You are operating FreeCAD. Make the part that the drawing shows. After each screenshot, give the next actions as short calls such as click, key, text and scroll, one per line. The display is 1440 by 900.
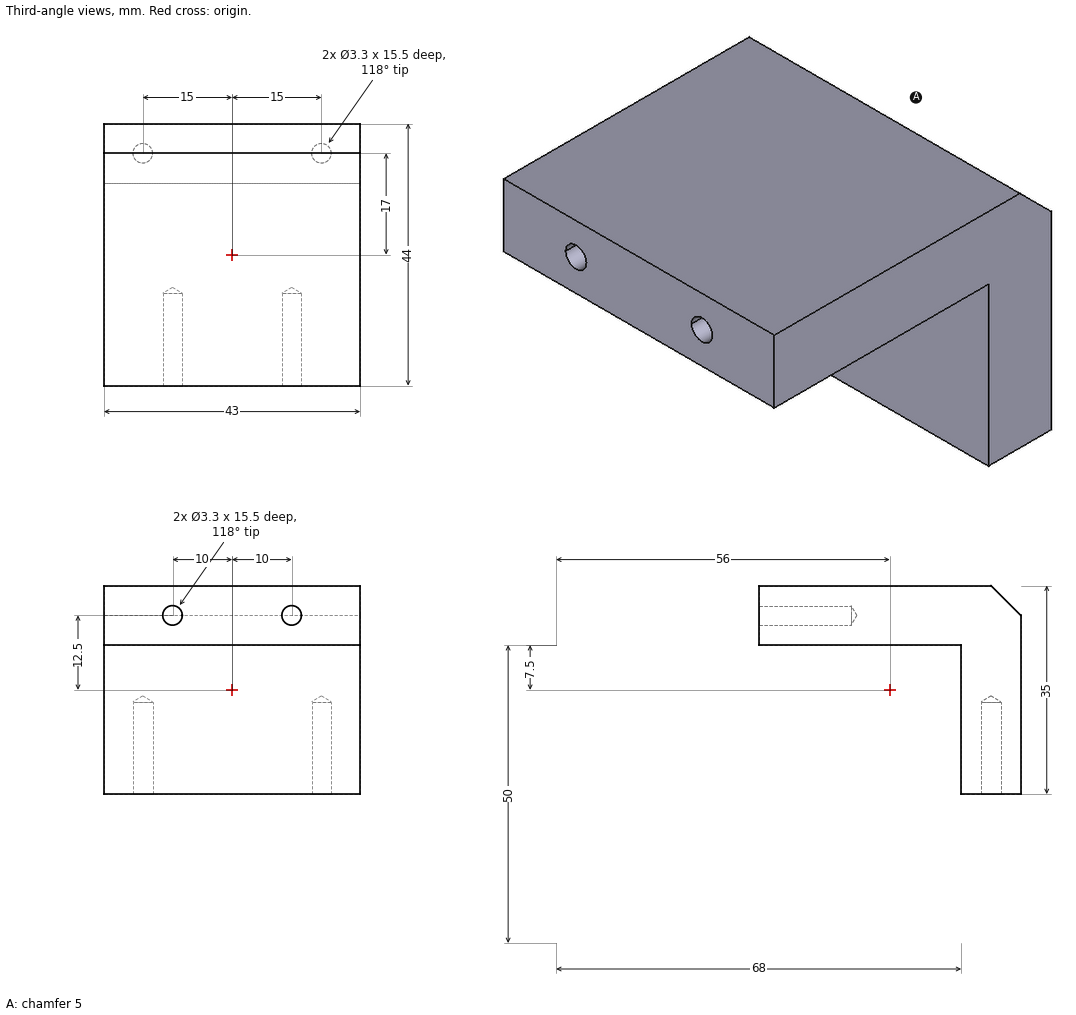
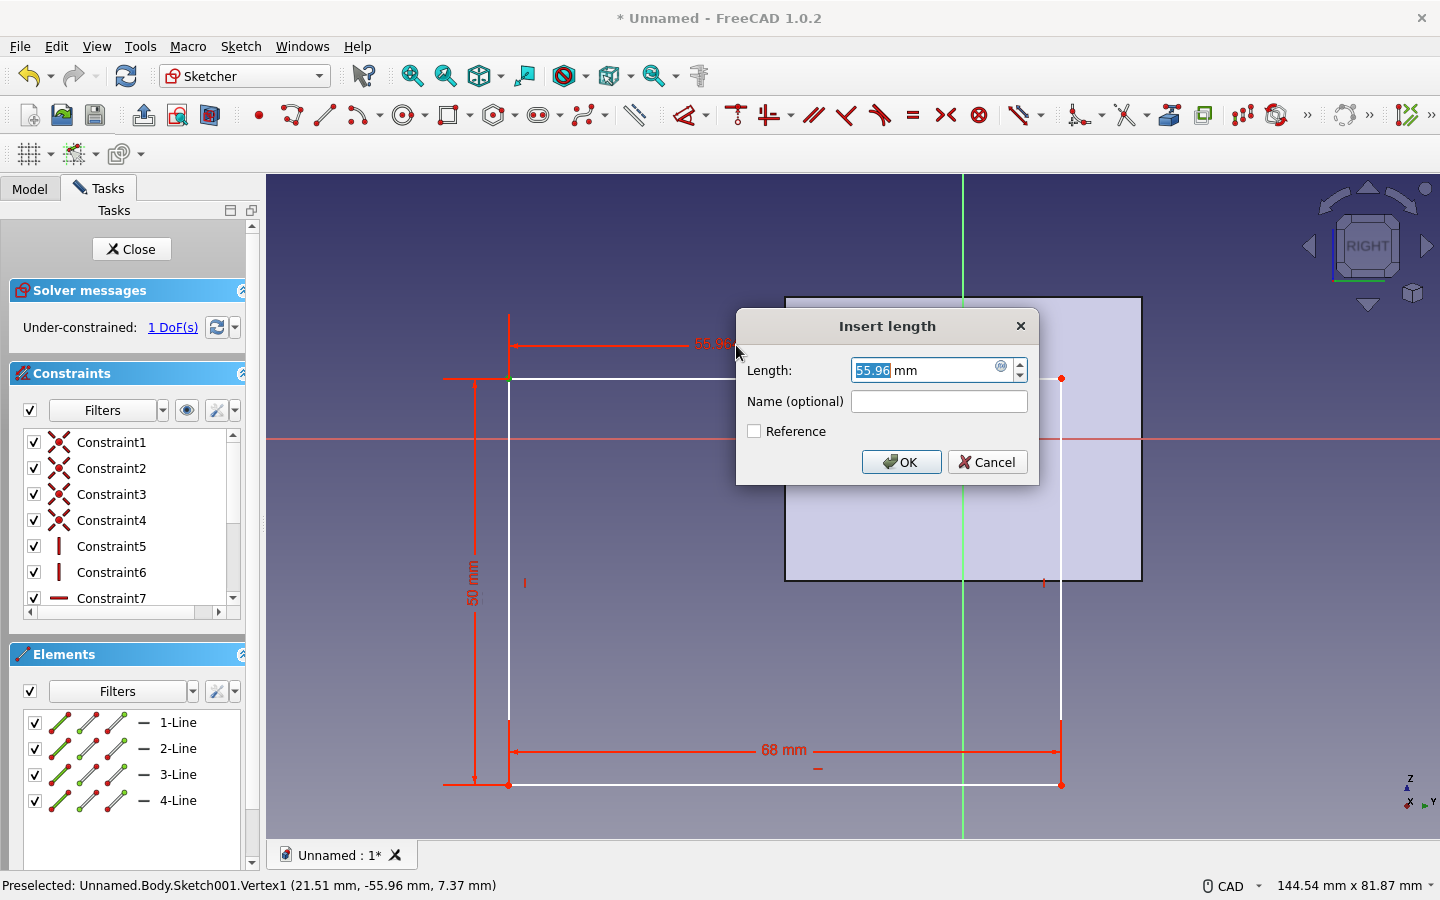
text(56)
key(Return)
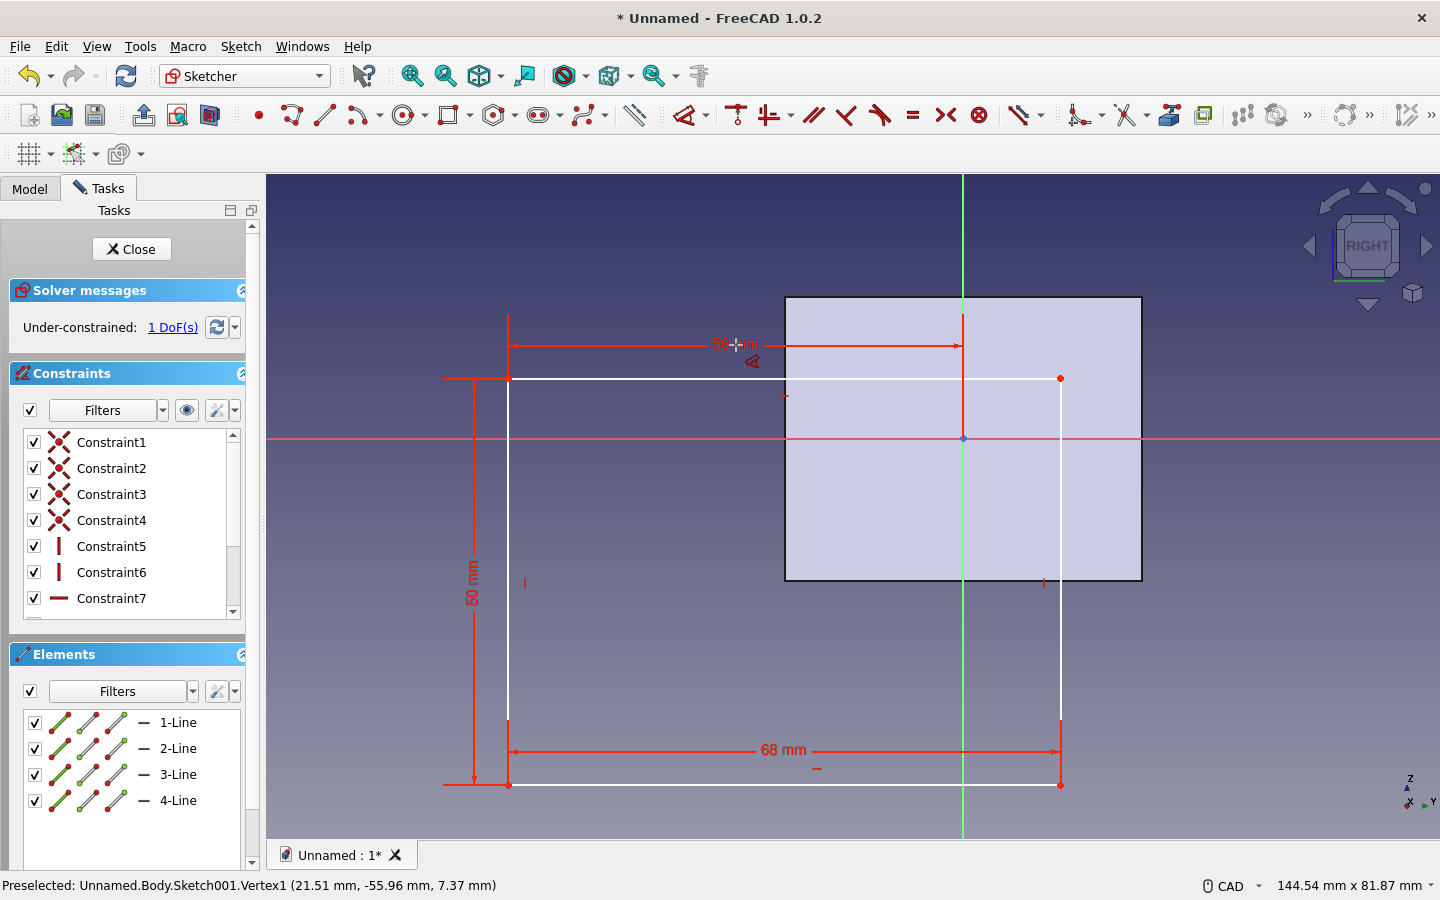
click(508, 379)
click(474, 409)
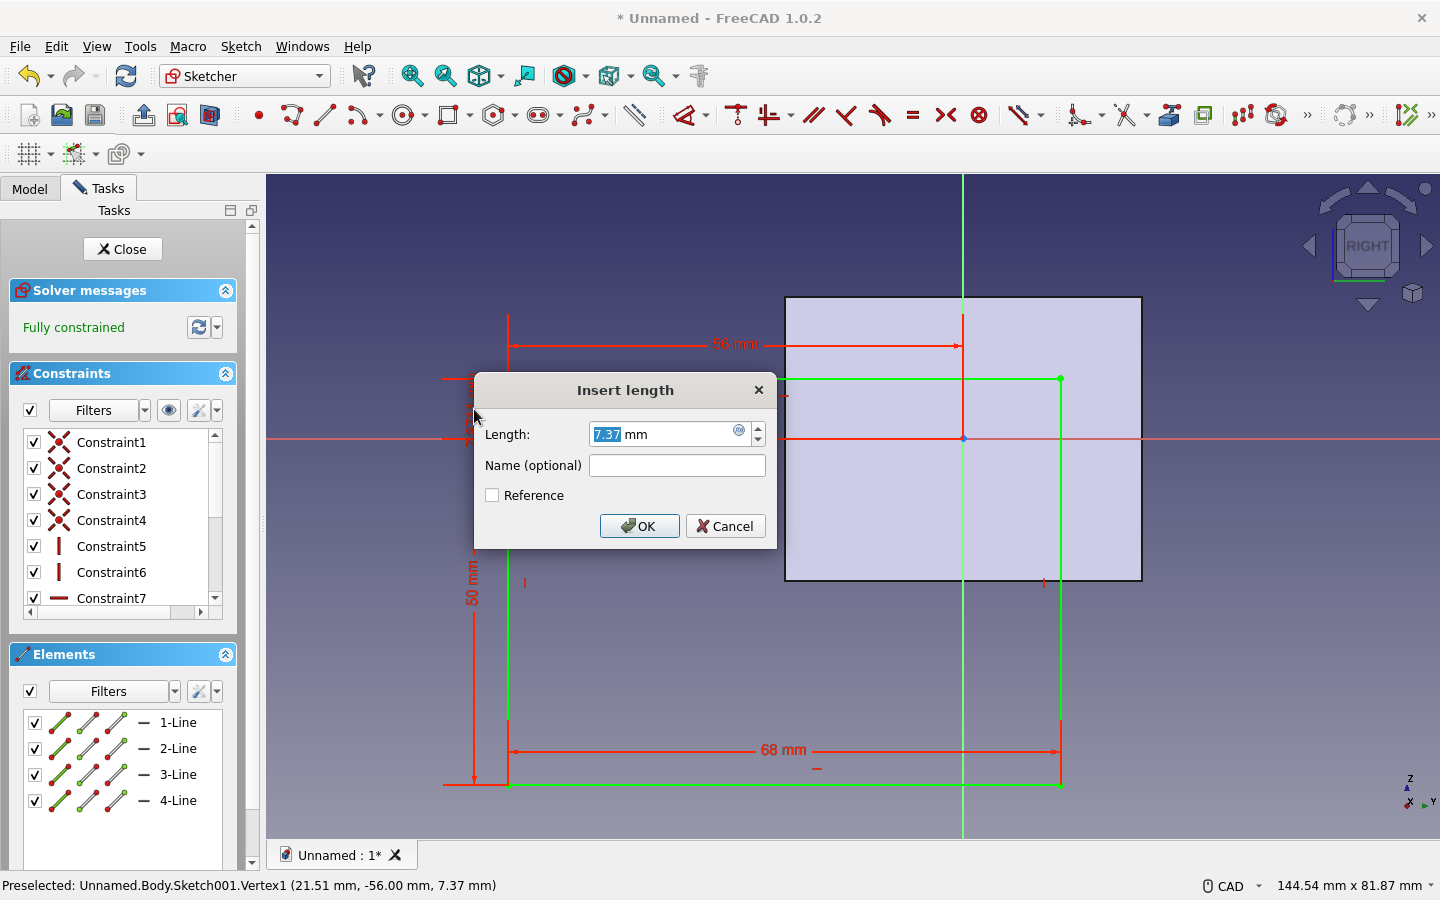
text(7.5)
key(Return)
key(Escape)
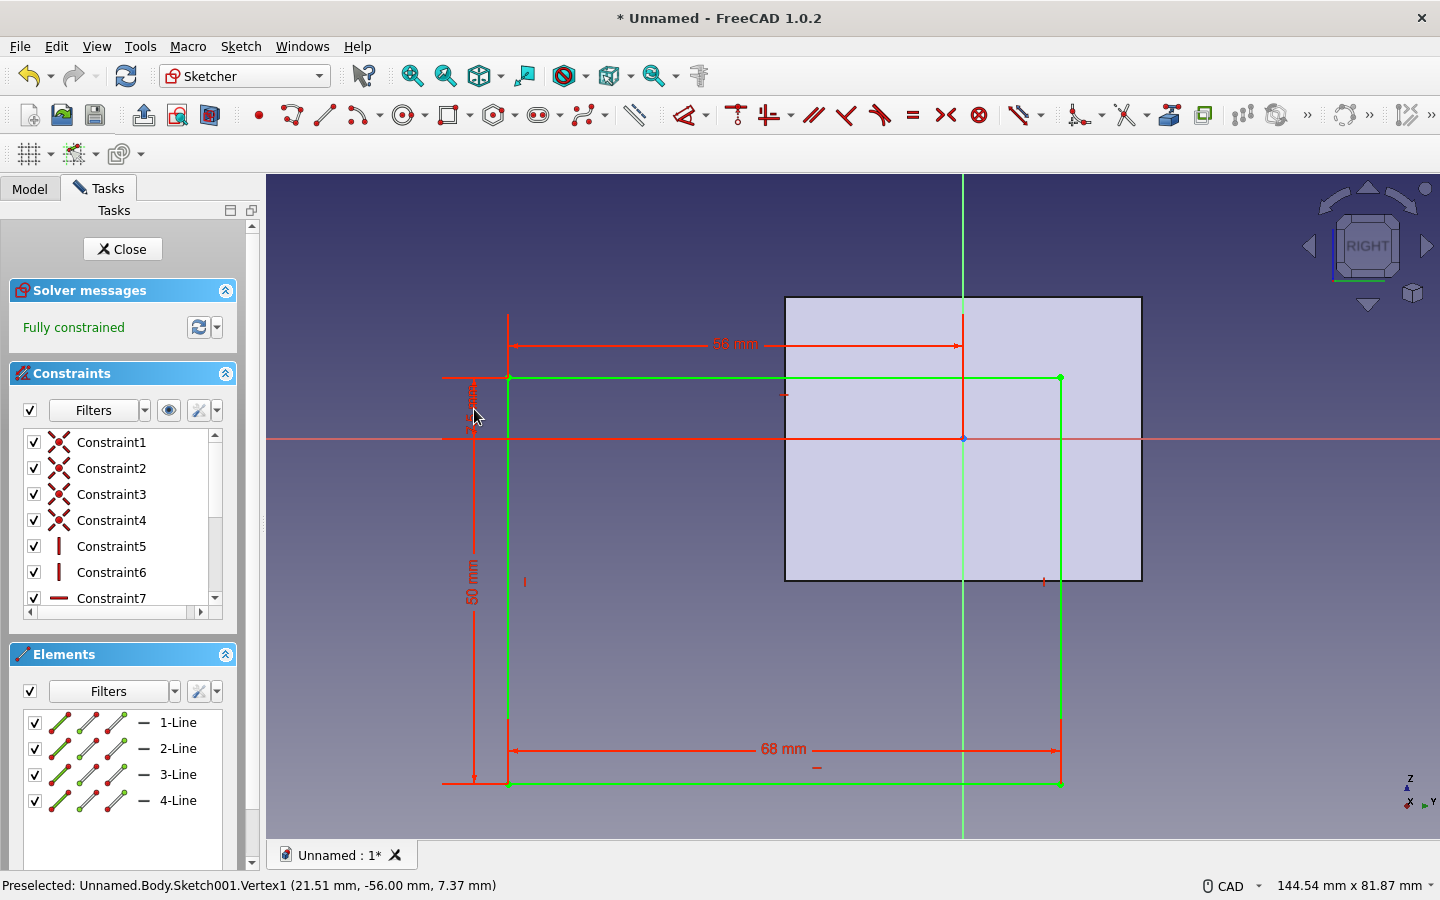
click(123, 249)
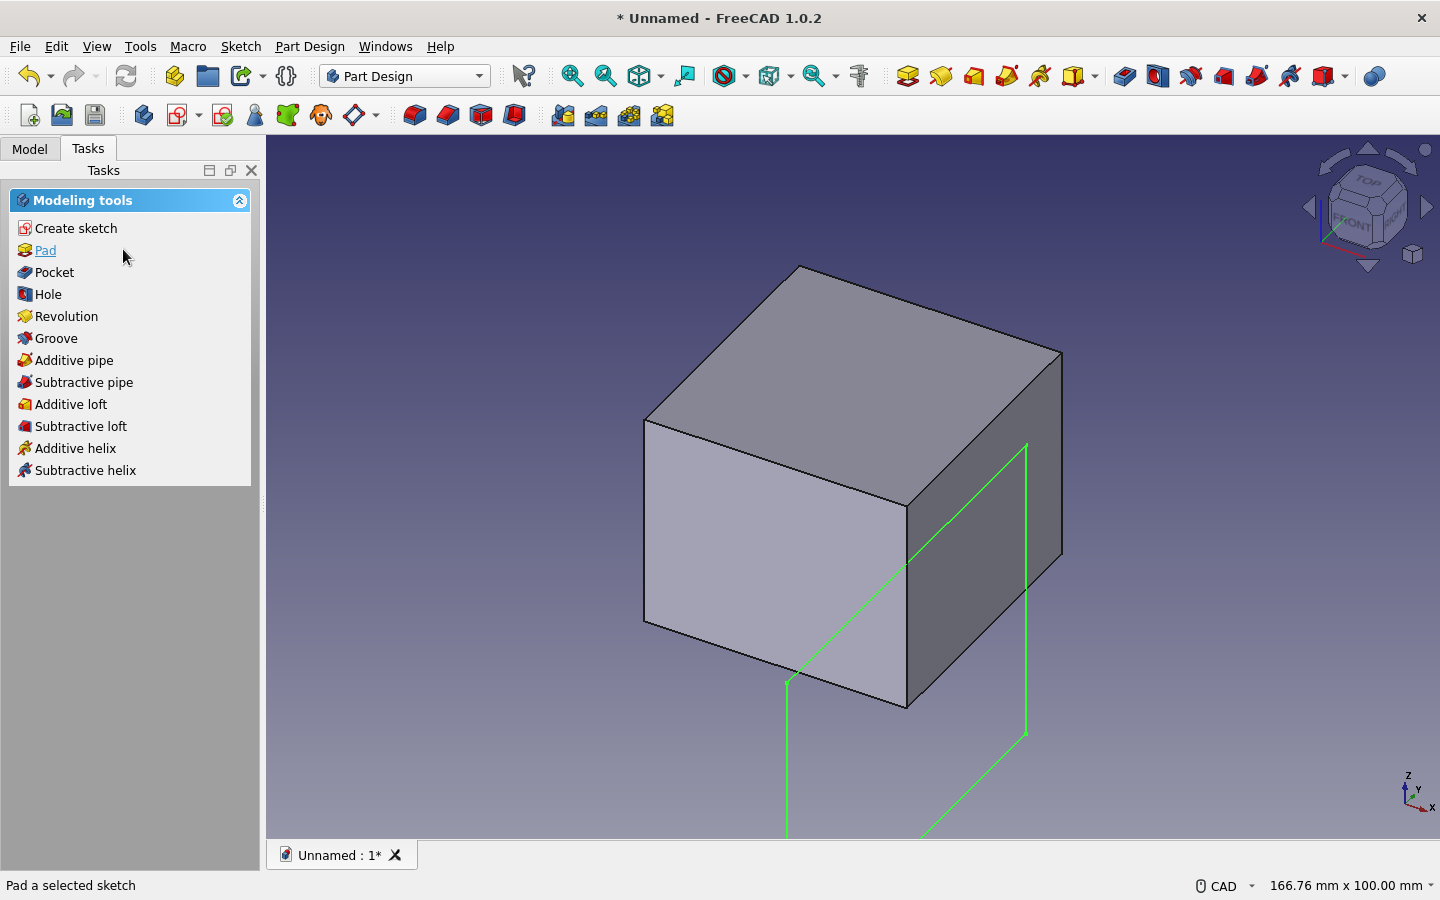
click(1125, 76)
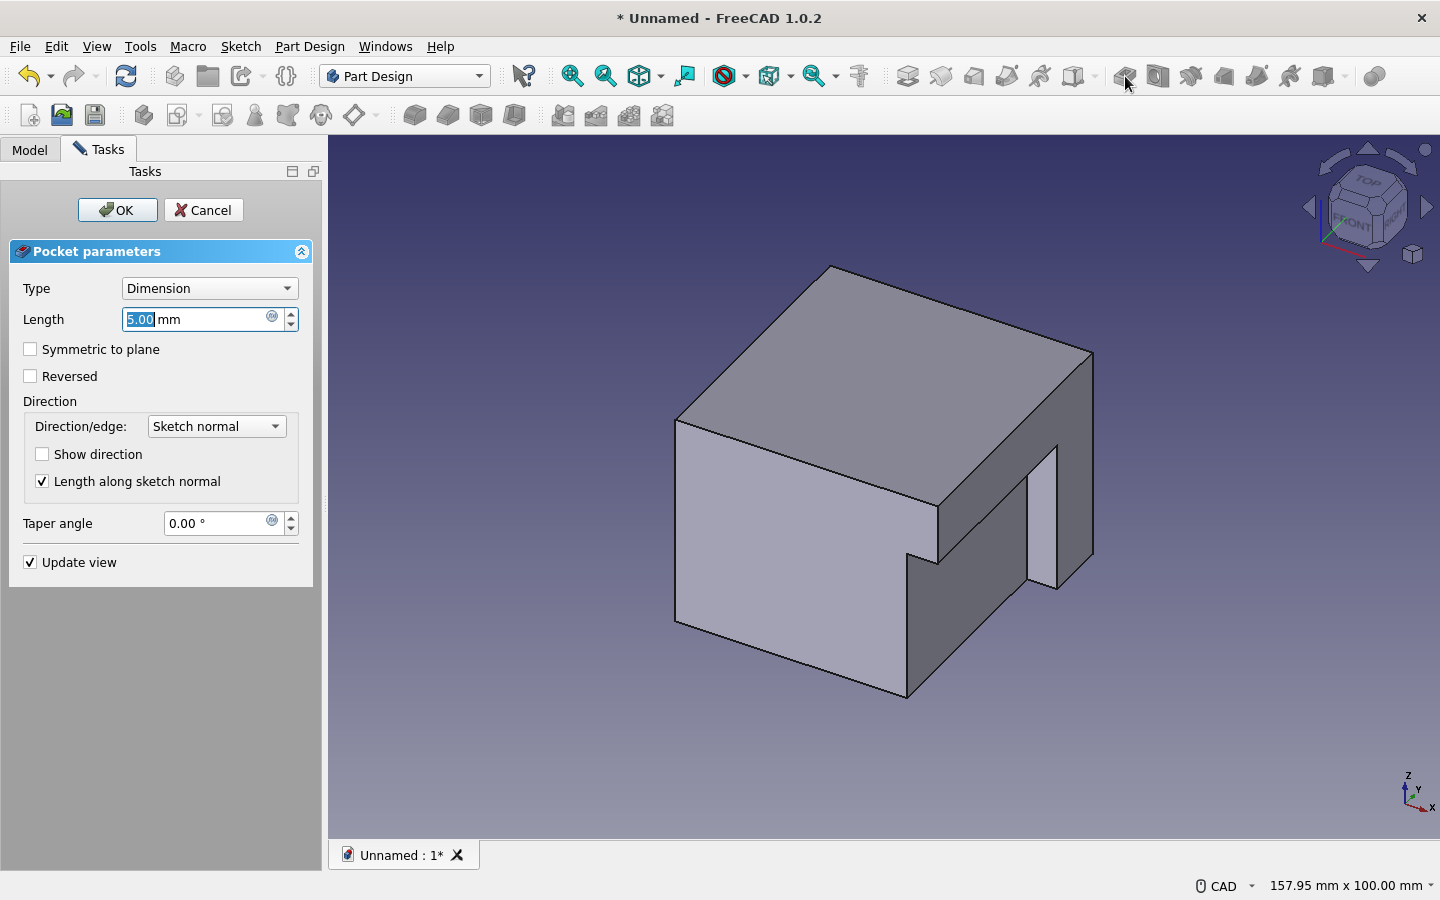
click(210, 288)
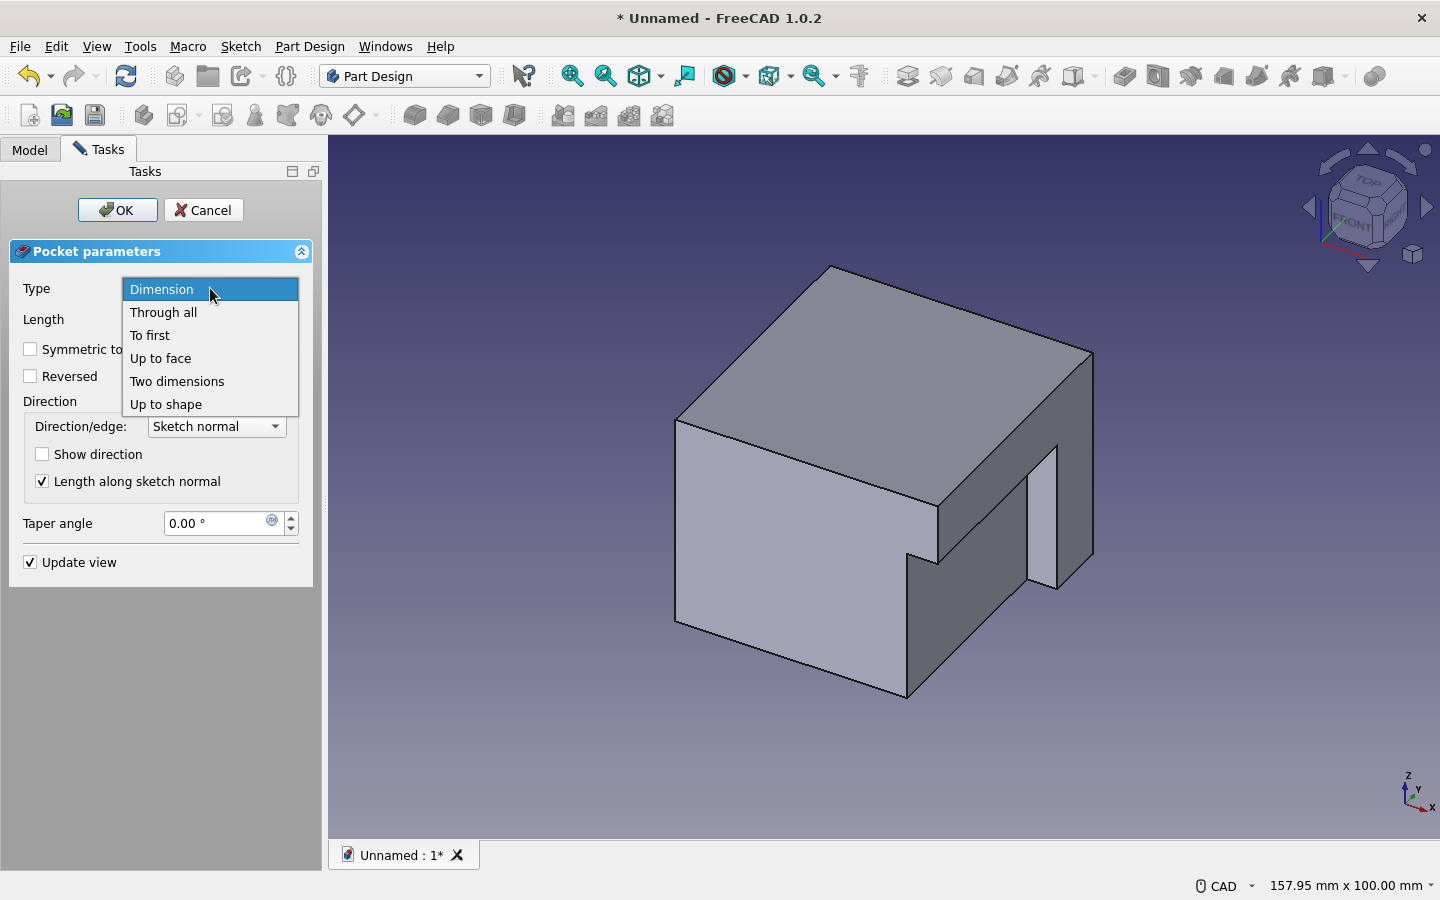
click(208, 312)